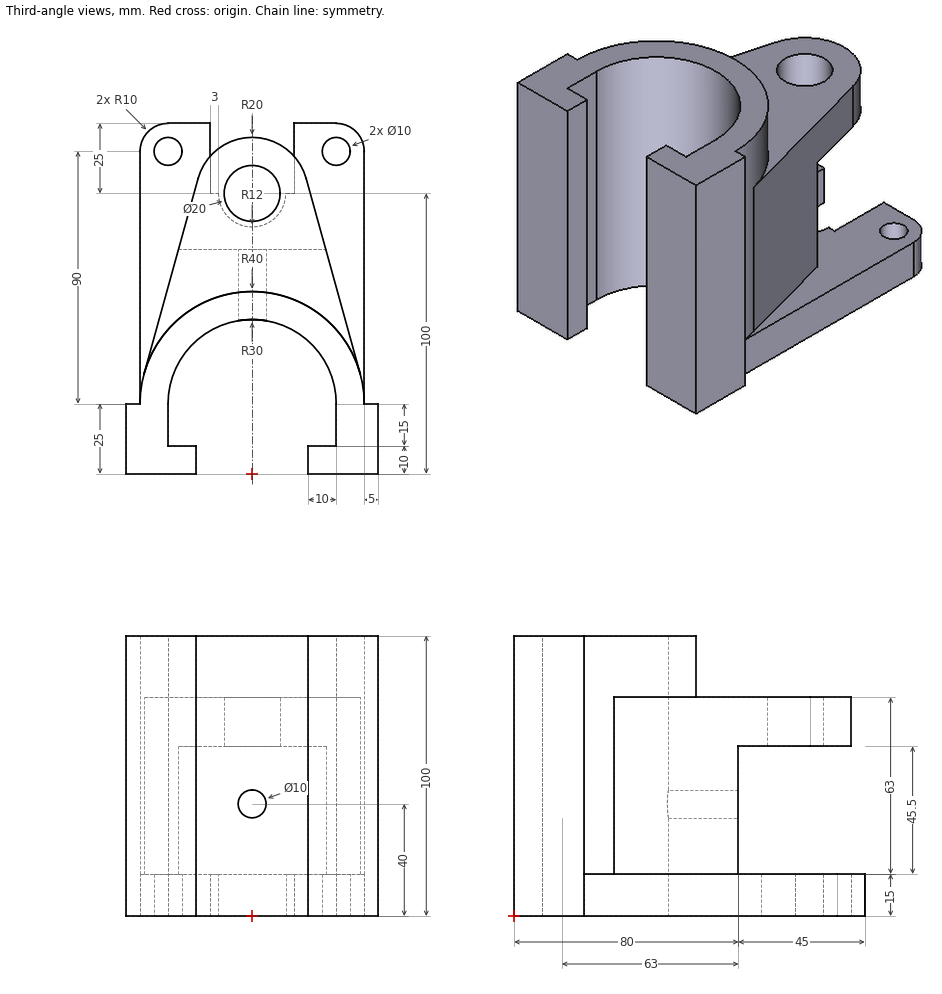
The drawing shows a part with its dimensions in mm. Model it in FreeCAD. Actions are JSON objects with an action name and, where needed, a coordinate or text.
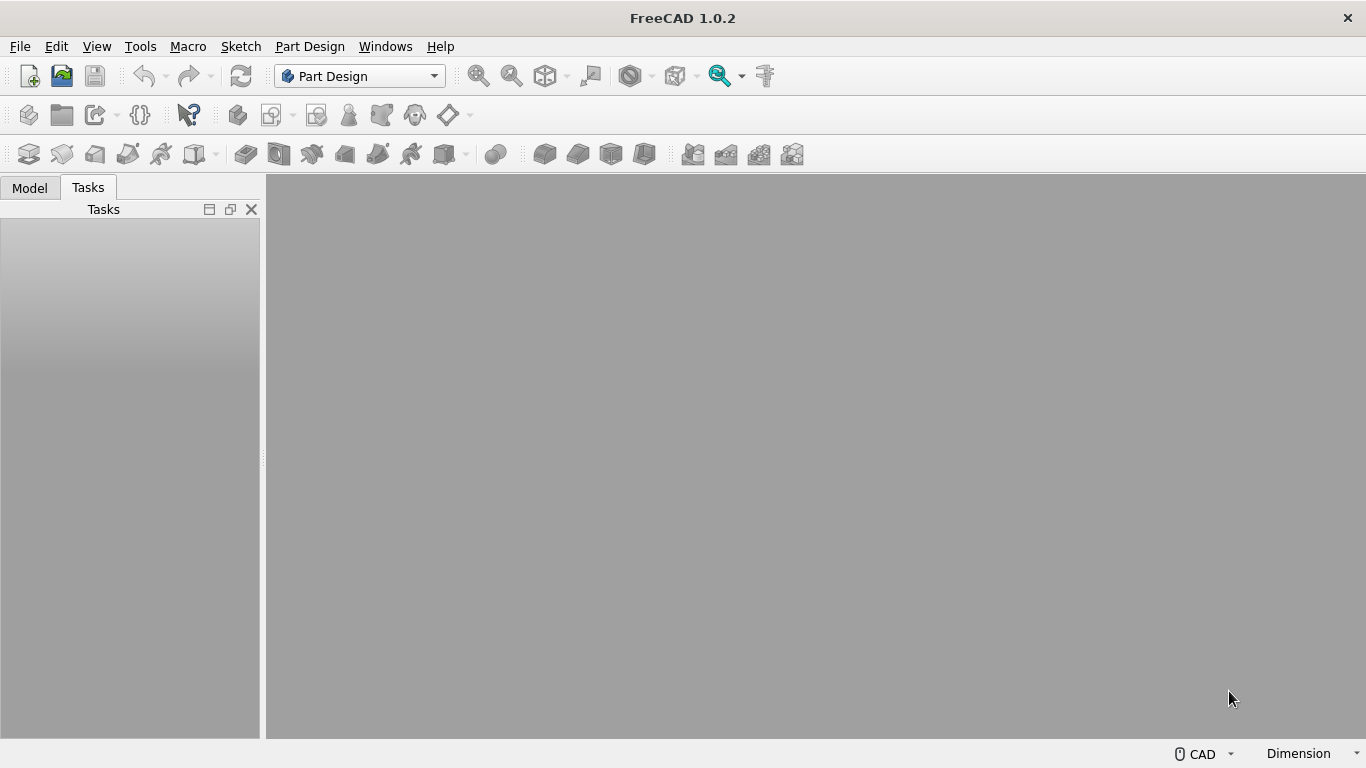
{"action": "key", "text": "ctrl+n"}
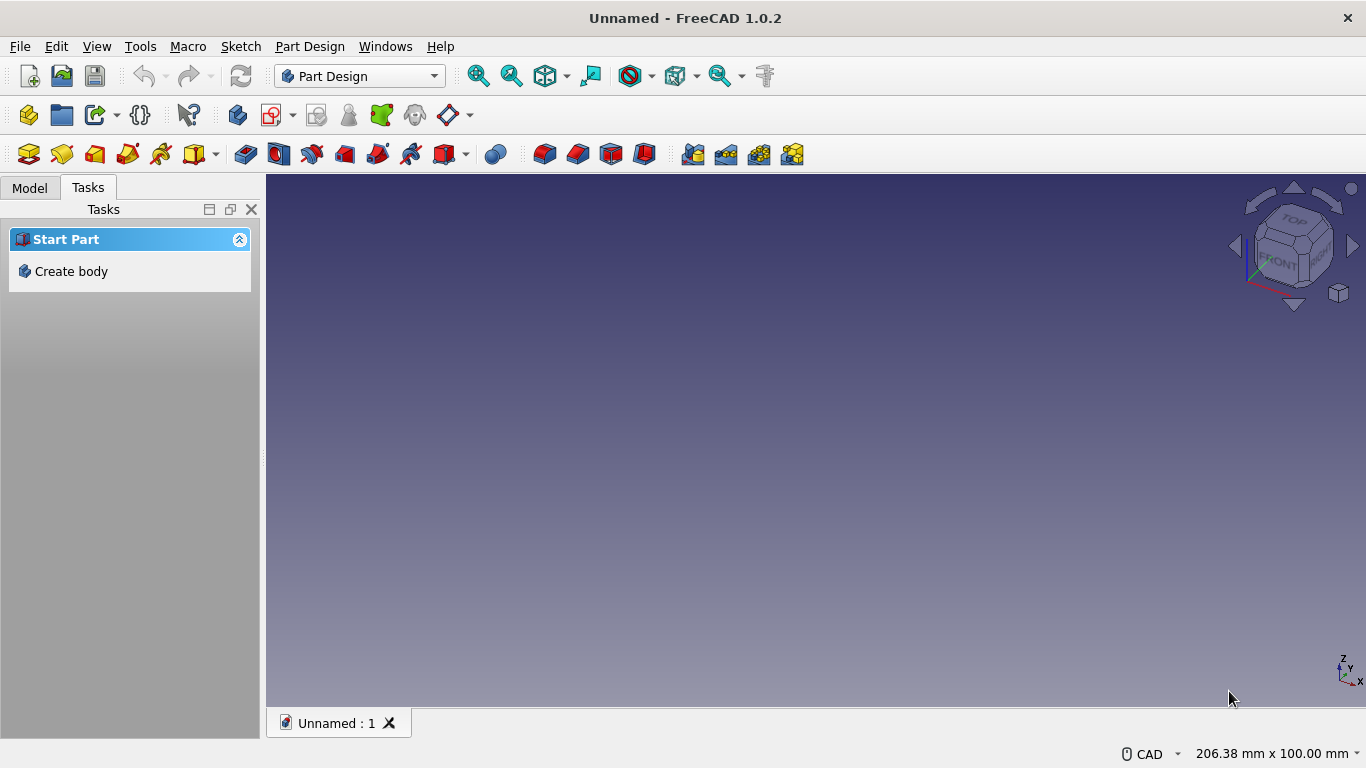
{"action": "left_click", "coordinate": [270, 116]}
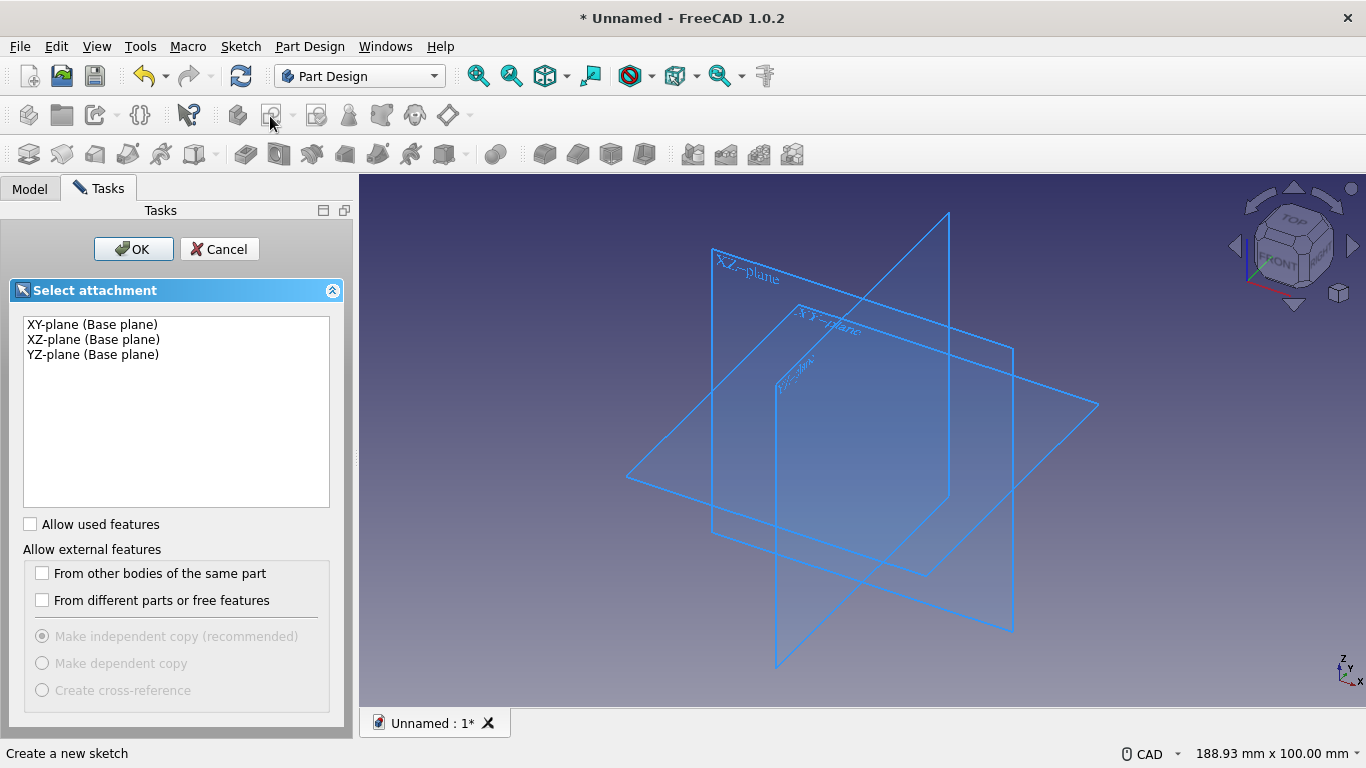
{"action": "left_click", "coordinate": [84, 324]}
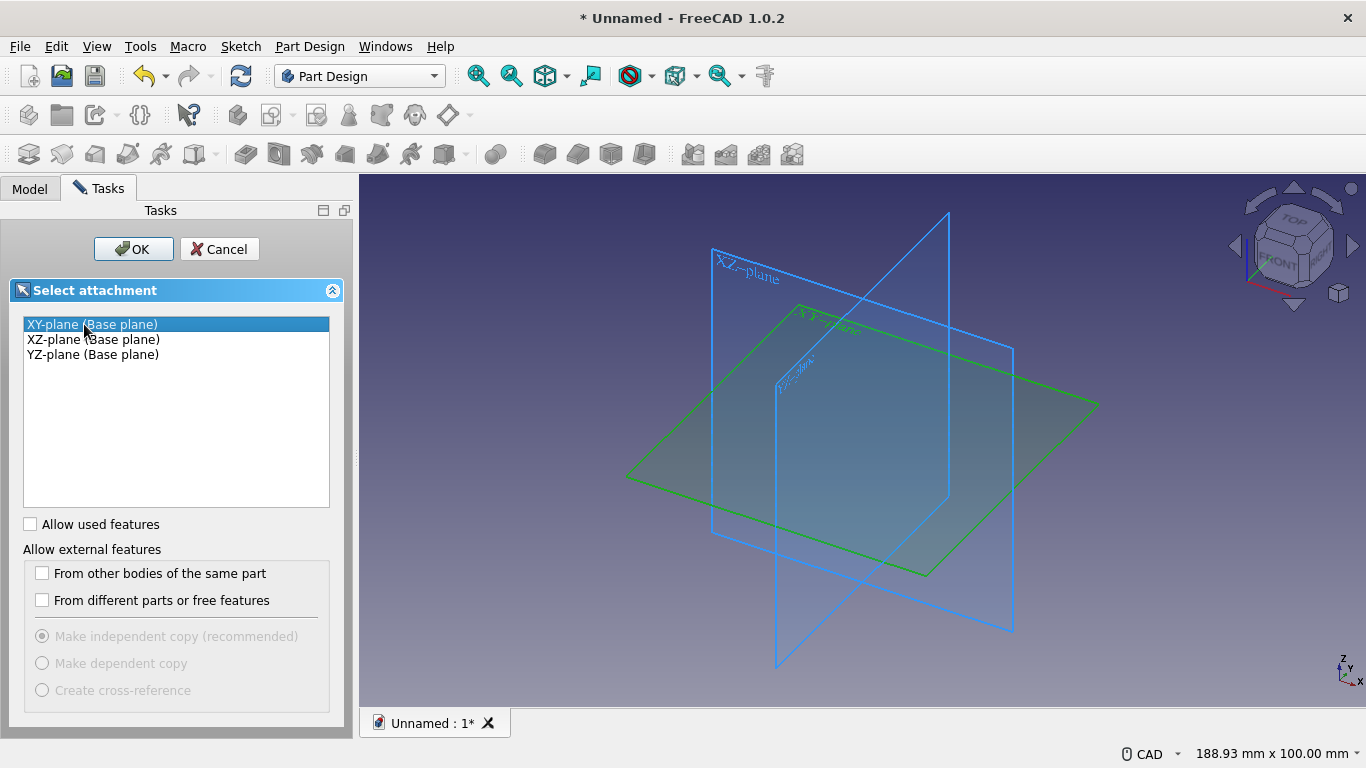
{"action": "left_click", "coordinate": [134, 249]}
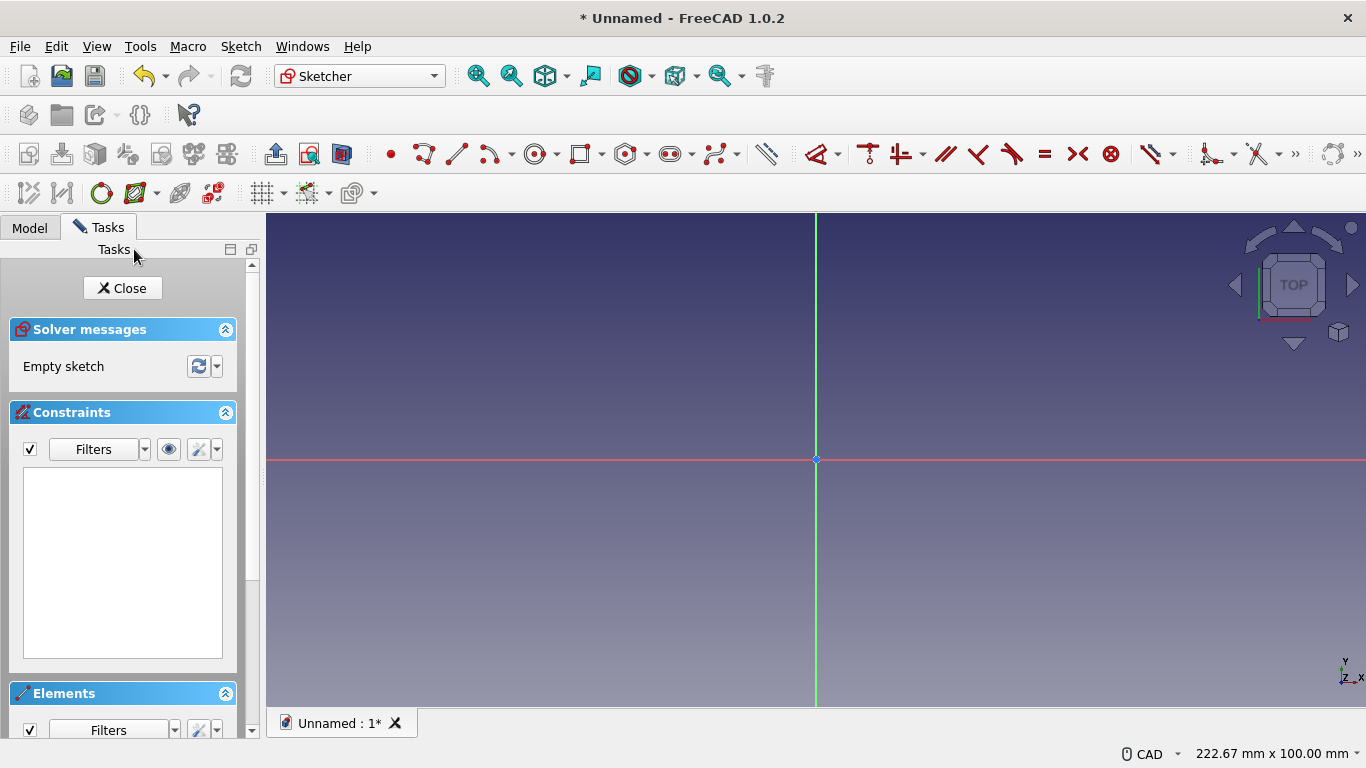
{"action": "scroll", "coordinate": [692, 679], "scroll_direction": "down", "scroll_amount": 4}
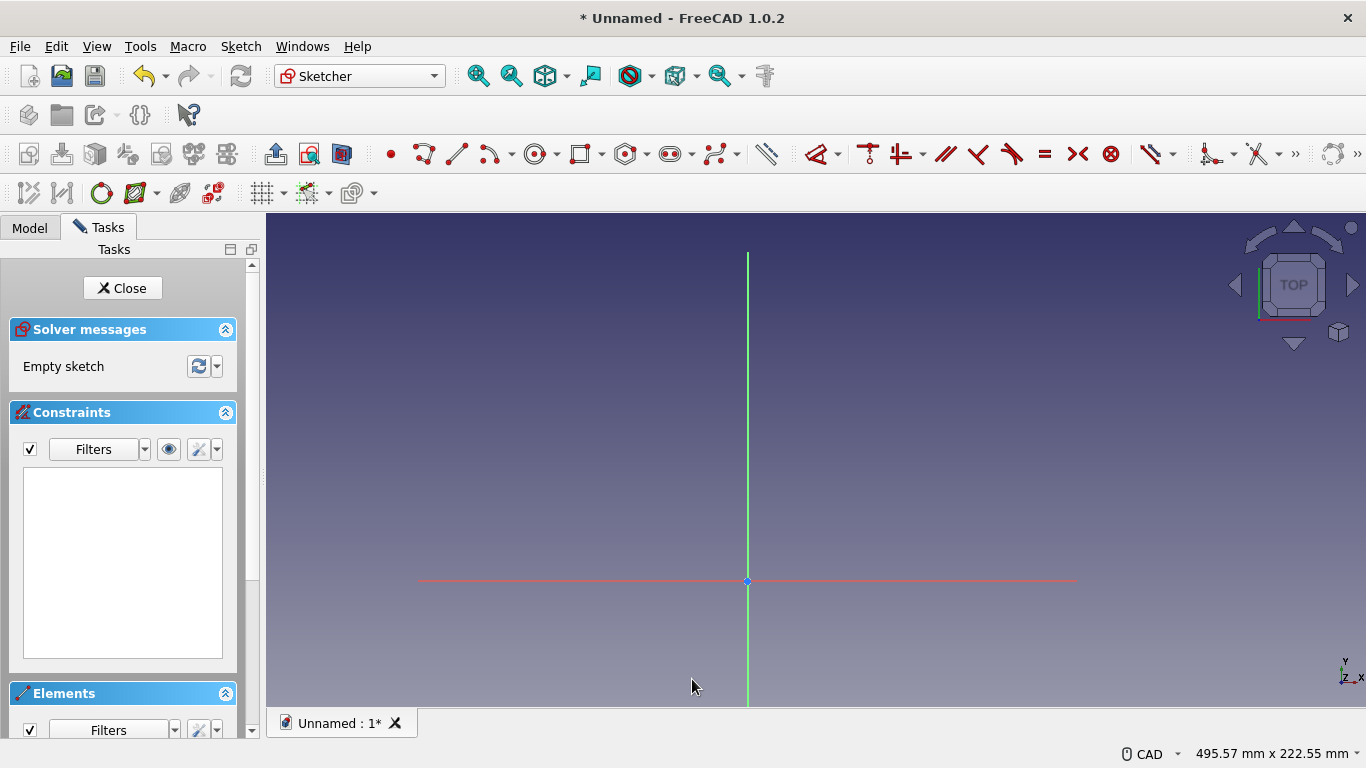
{"action": "key", "text": "g m"}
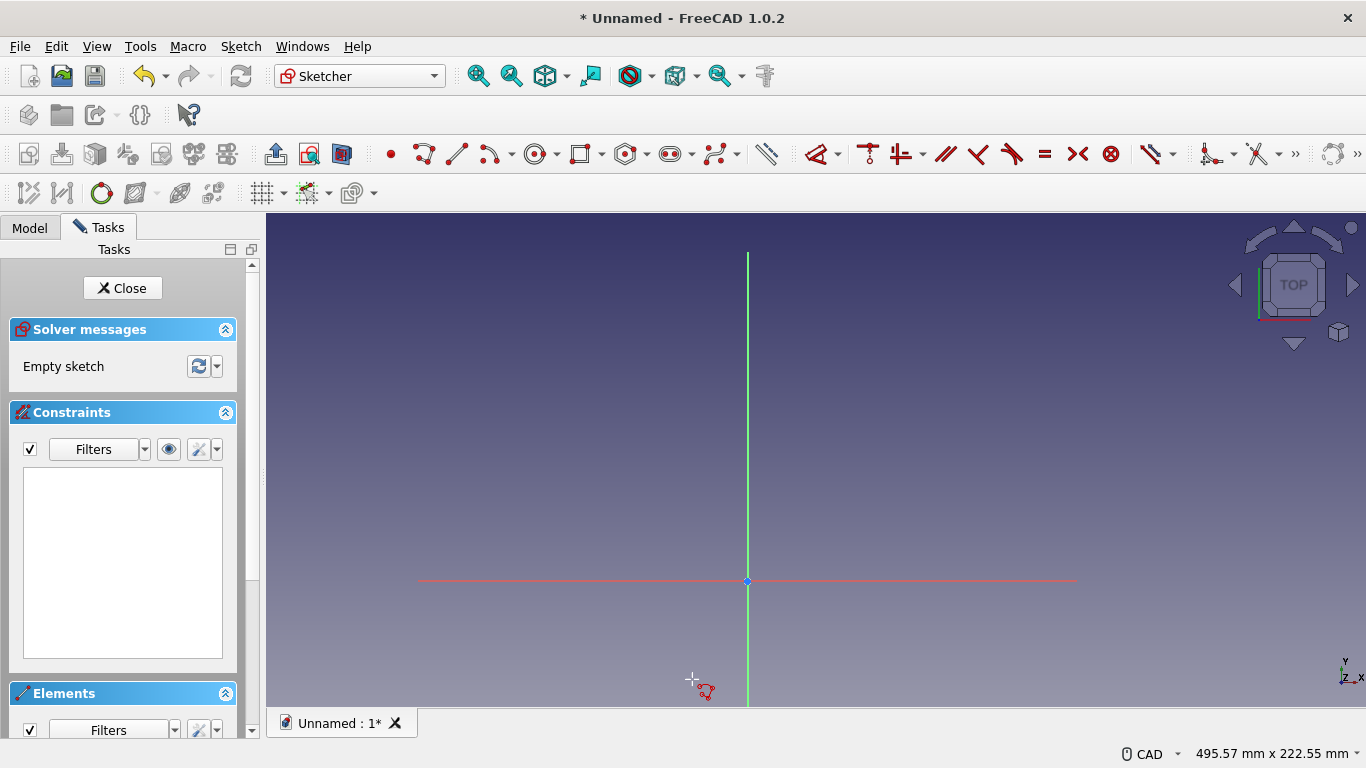
{"action": "left_click", "coordinate": [721, 359]}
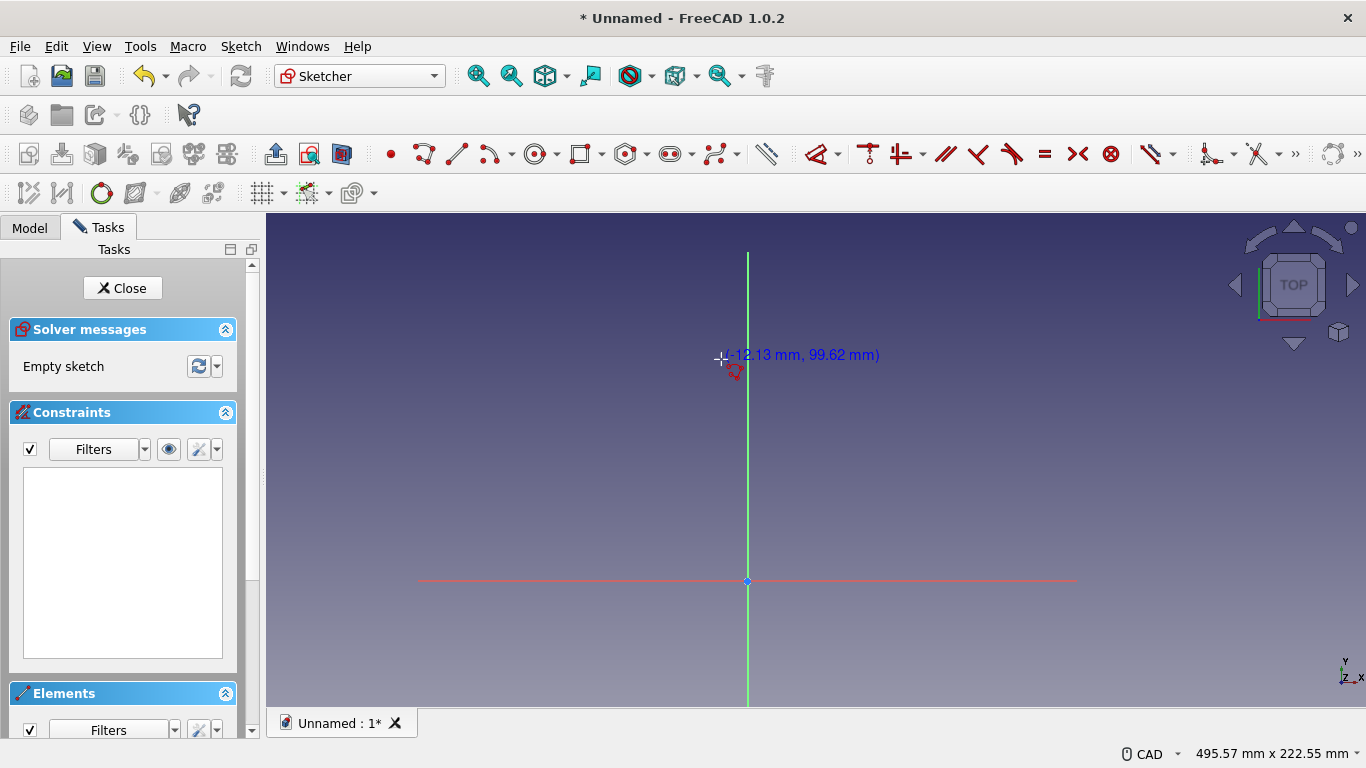
{"action": "scroll", "coordinate": [715, 359], "scroll_direction": "up", "scroll_amount": 5}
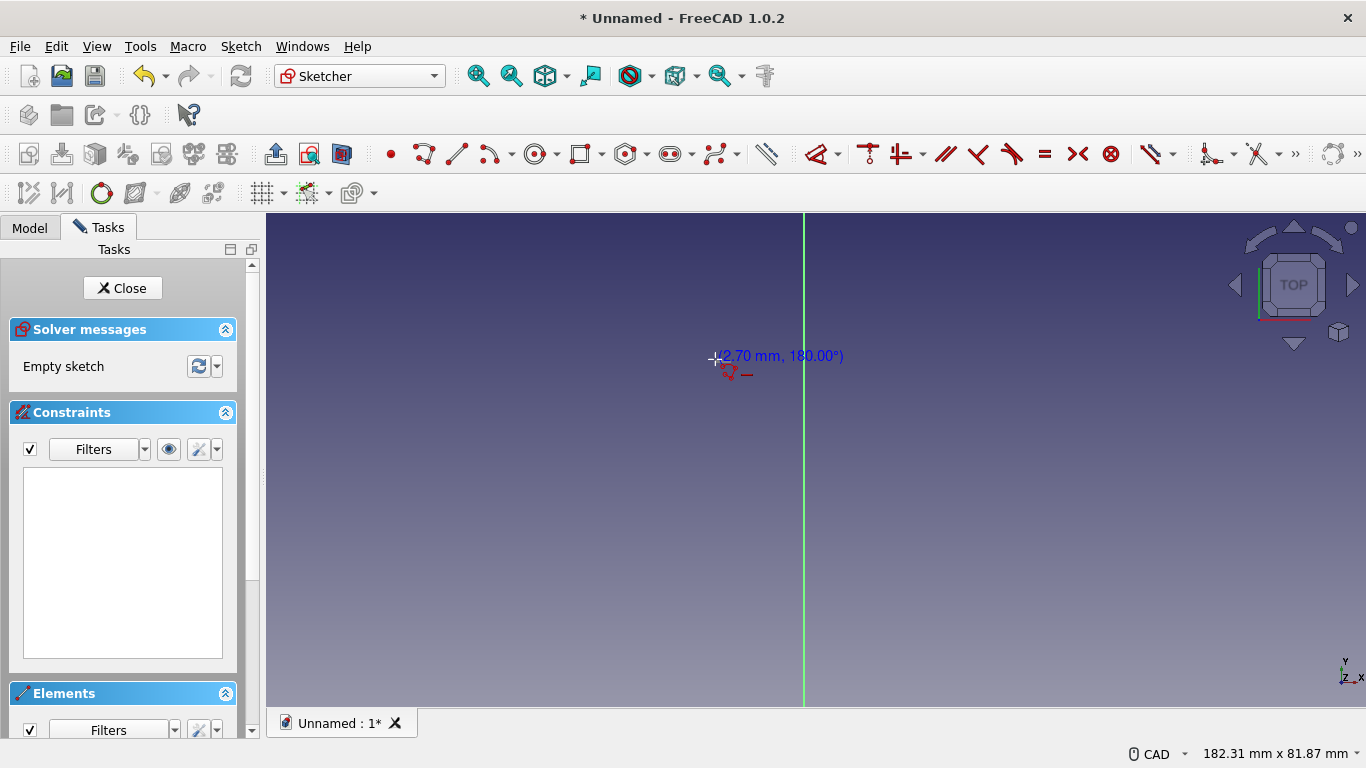
{"action": "left_click", "coordinate": [713, 358]}